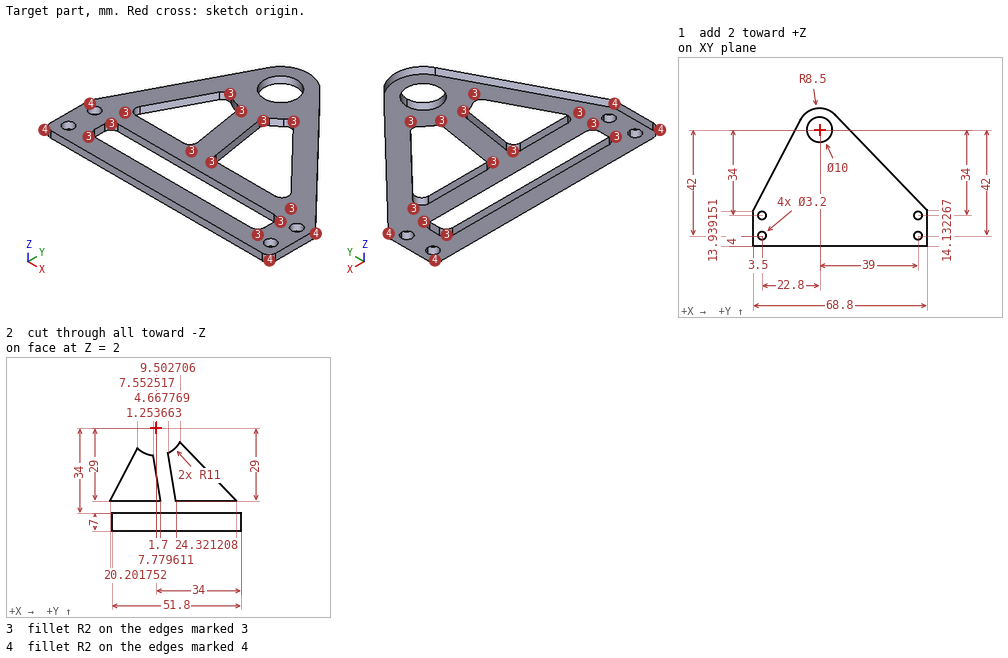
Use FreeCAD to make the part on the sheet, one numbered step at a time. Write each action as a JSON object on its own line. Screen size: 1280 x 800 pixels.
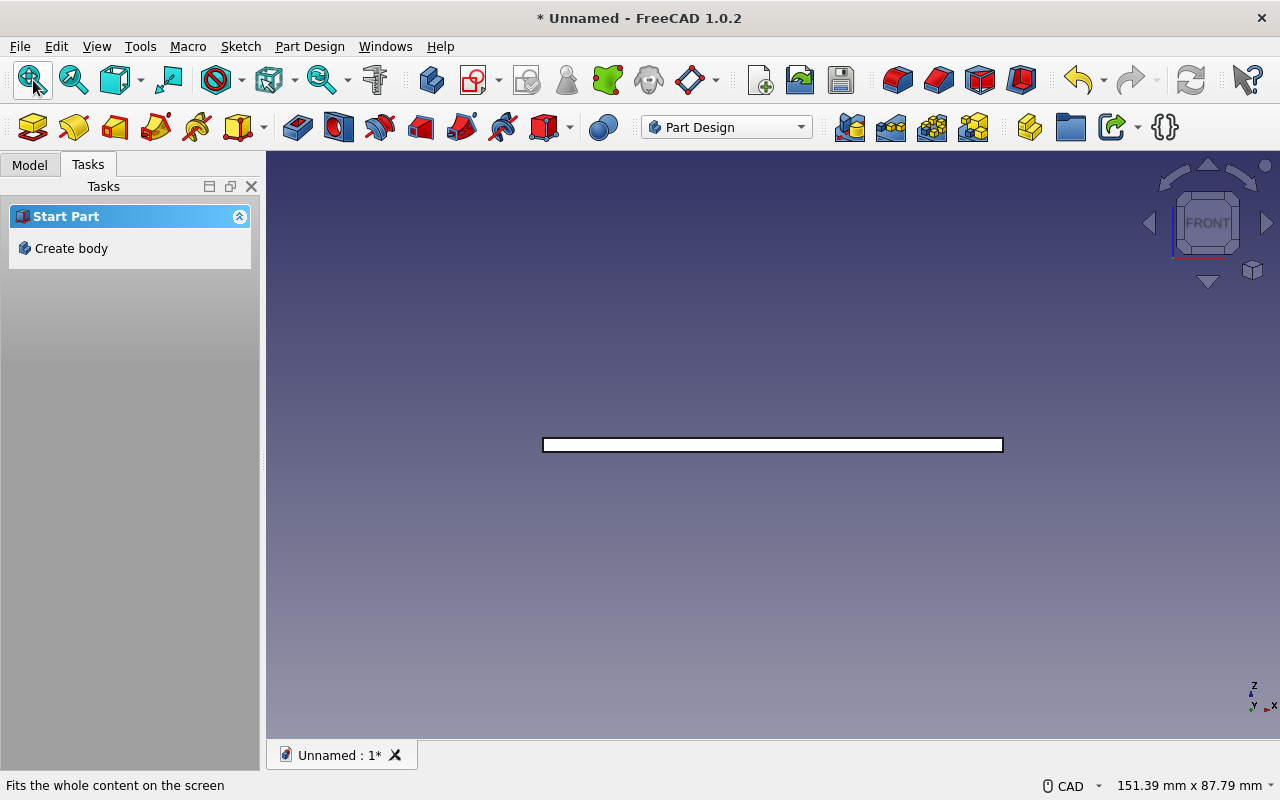
{"action": "scroll", "coordinate": [600, 444], "scroll_direction": "up", "scroll_amount": 6}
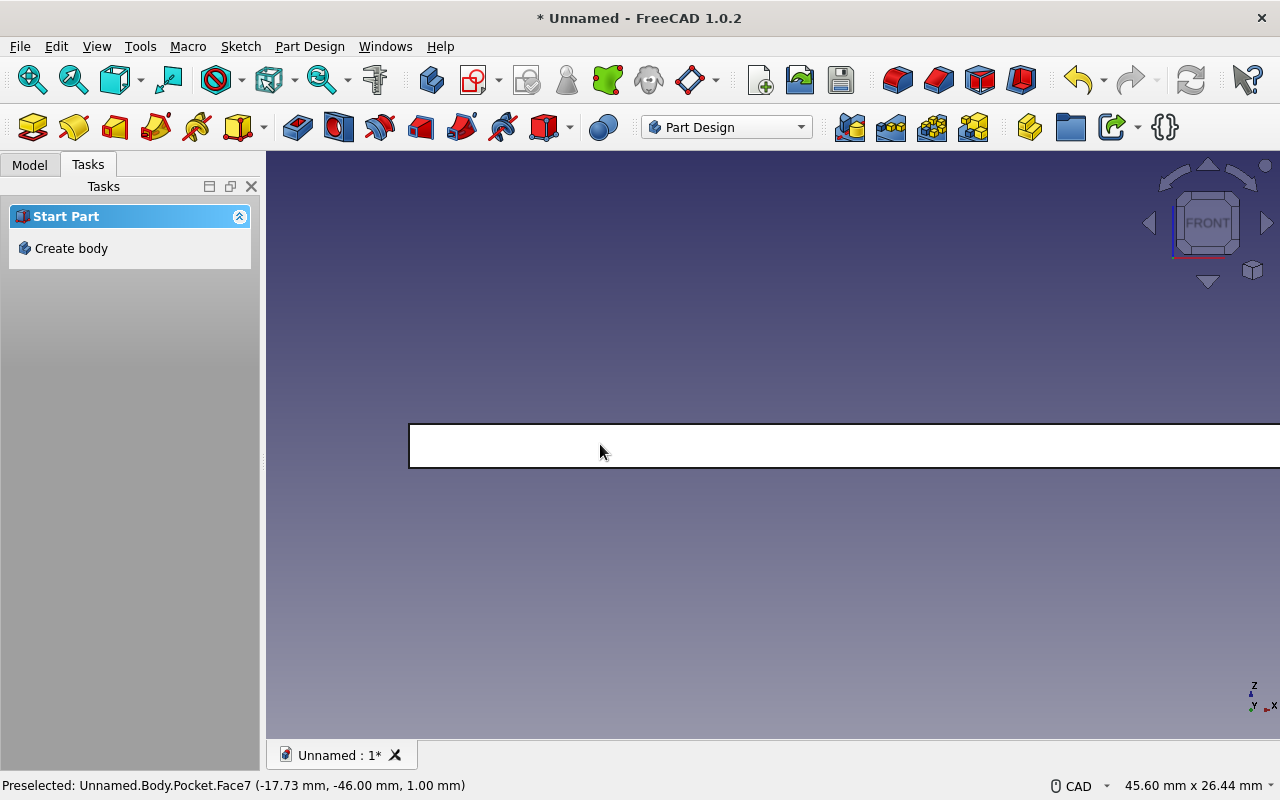
{"action": "left_click", "coordinate": [33, 80]}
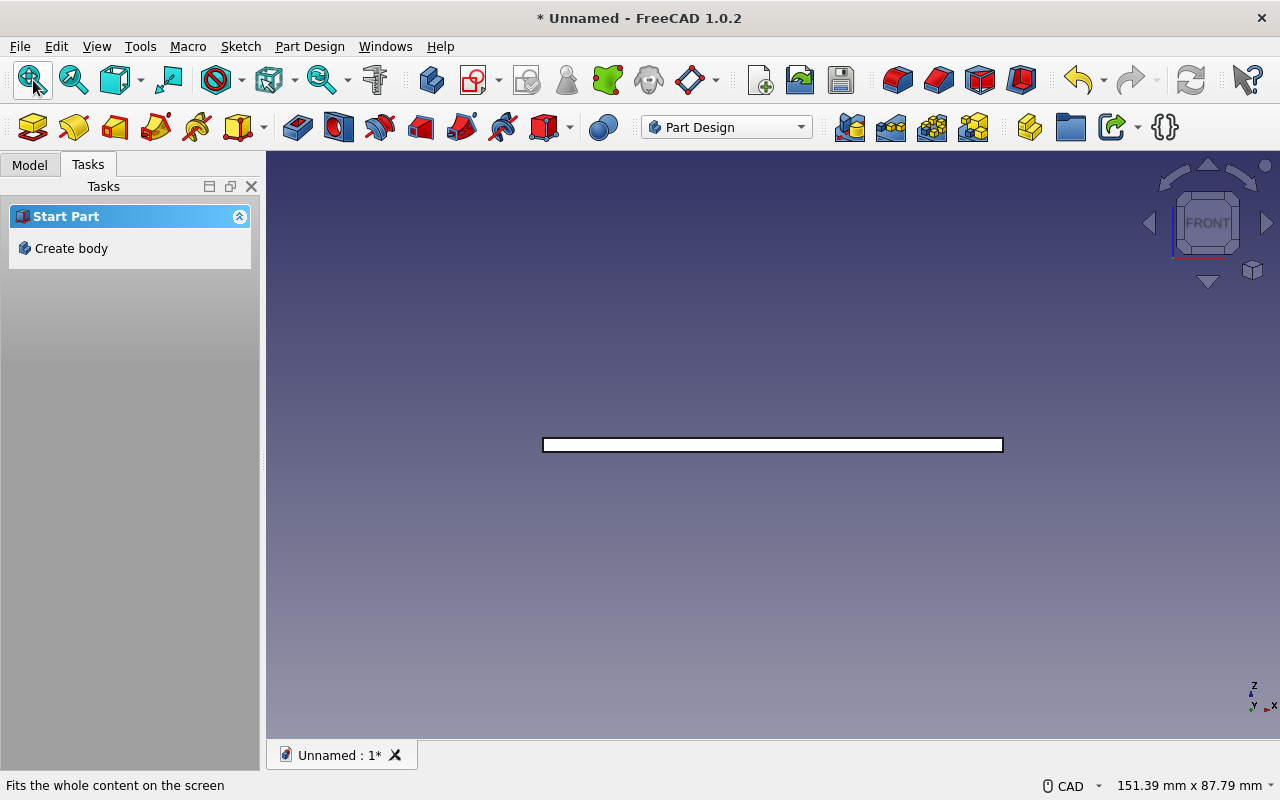
{"action": "key", "text": "3"}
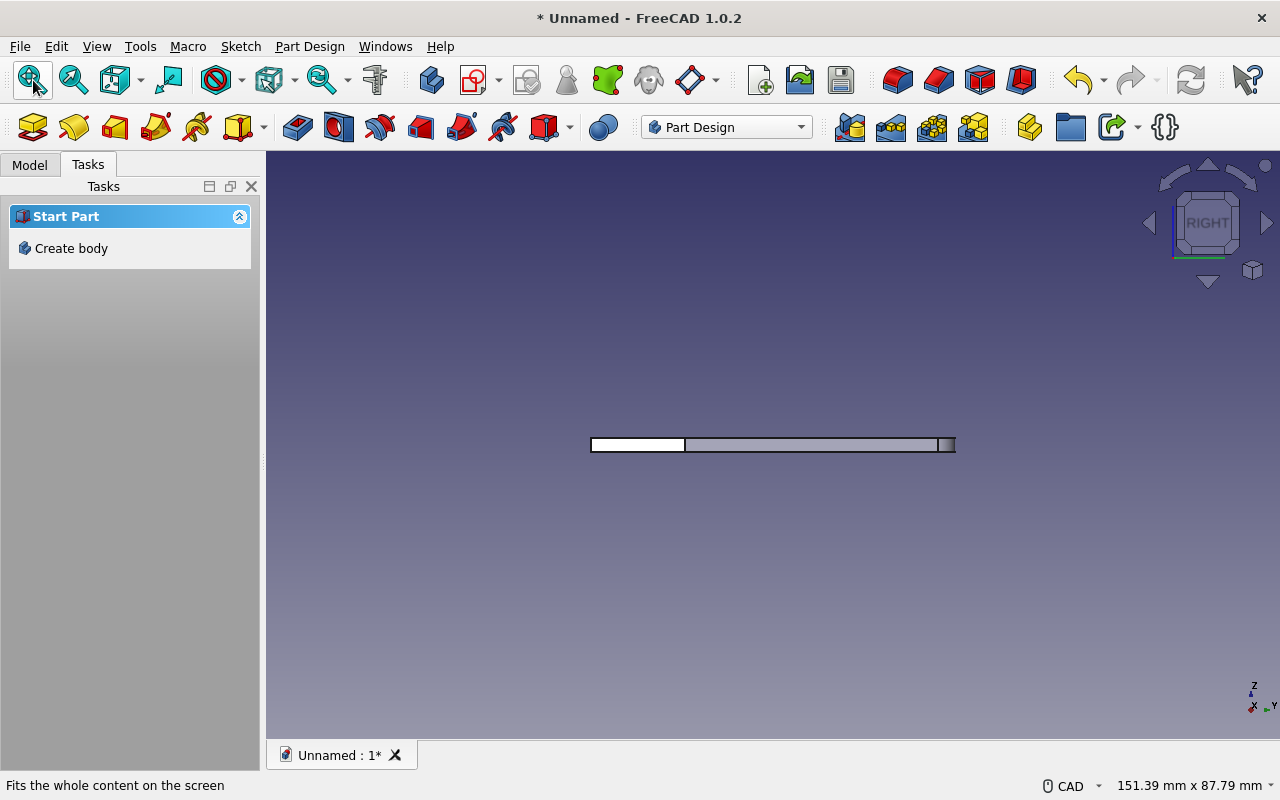
{"action": "key", "text": "v f"}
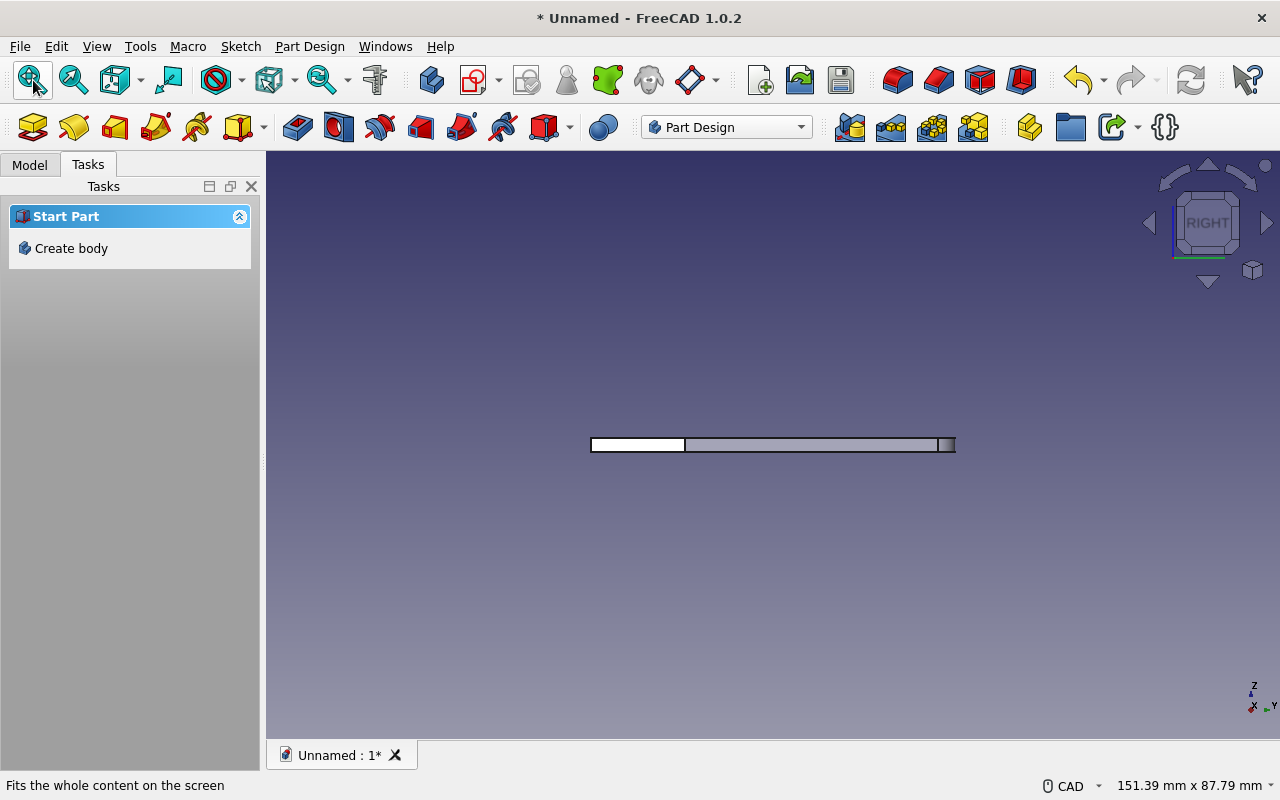
{"action": "scroll", "coordinate": [624, 444], "scroll_direction": "up", "scroll_amount": 6}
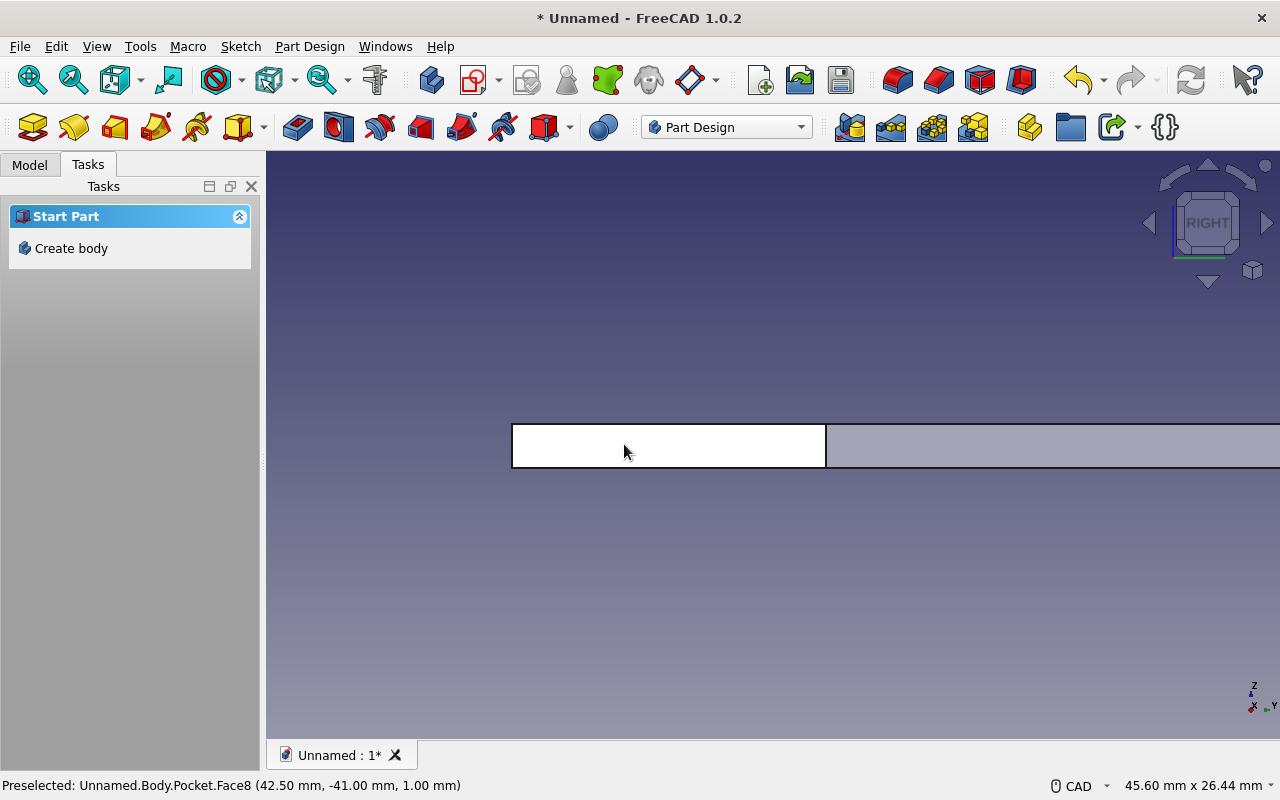
{"action": "left_click", "coordinate": [33, 80]}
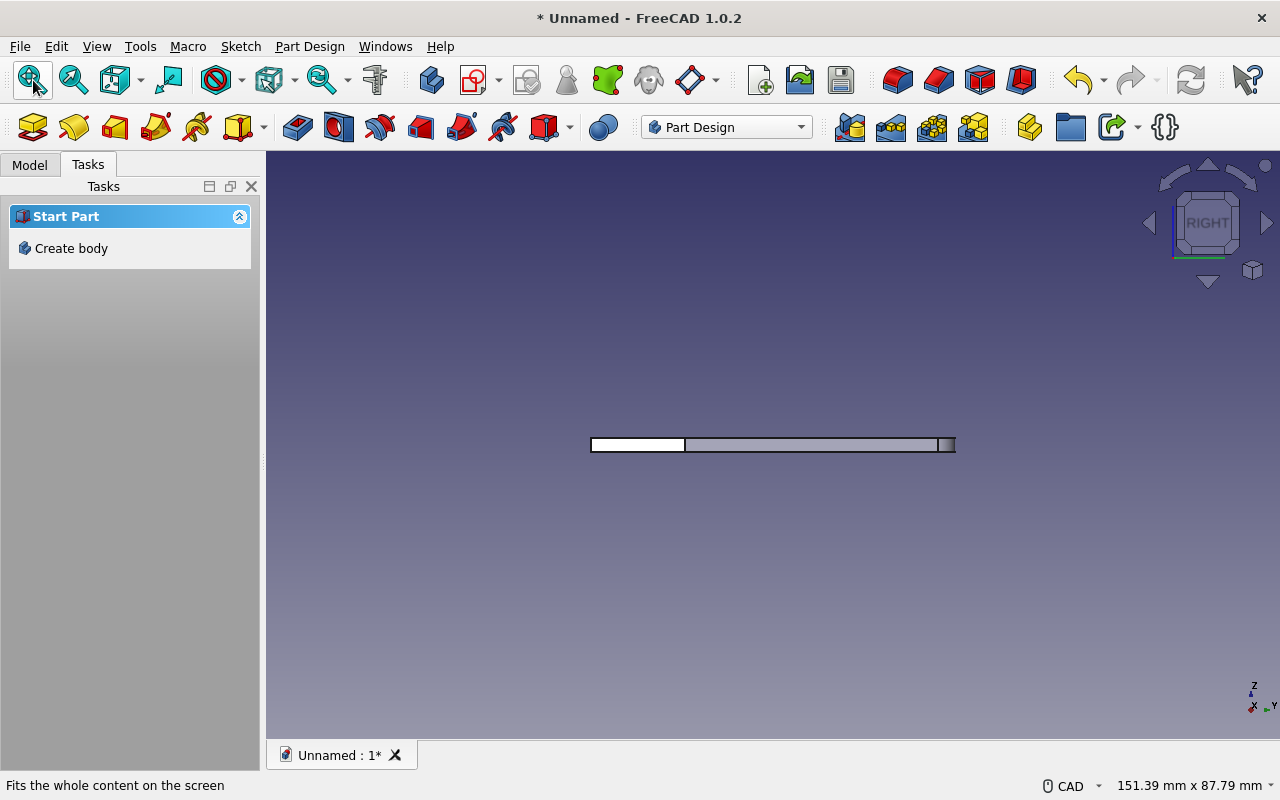
{"action": "key", "text": "5"}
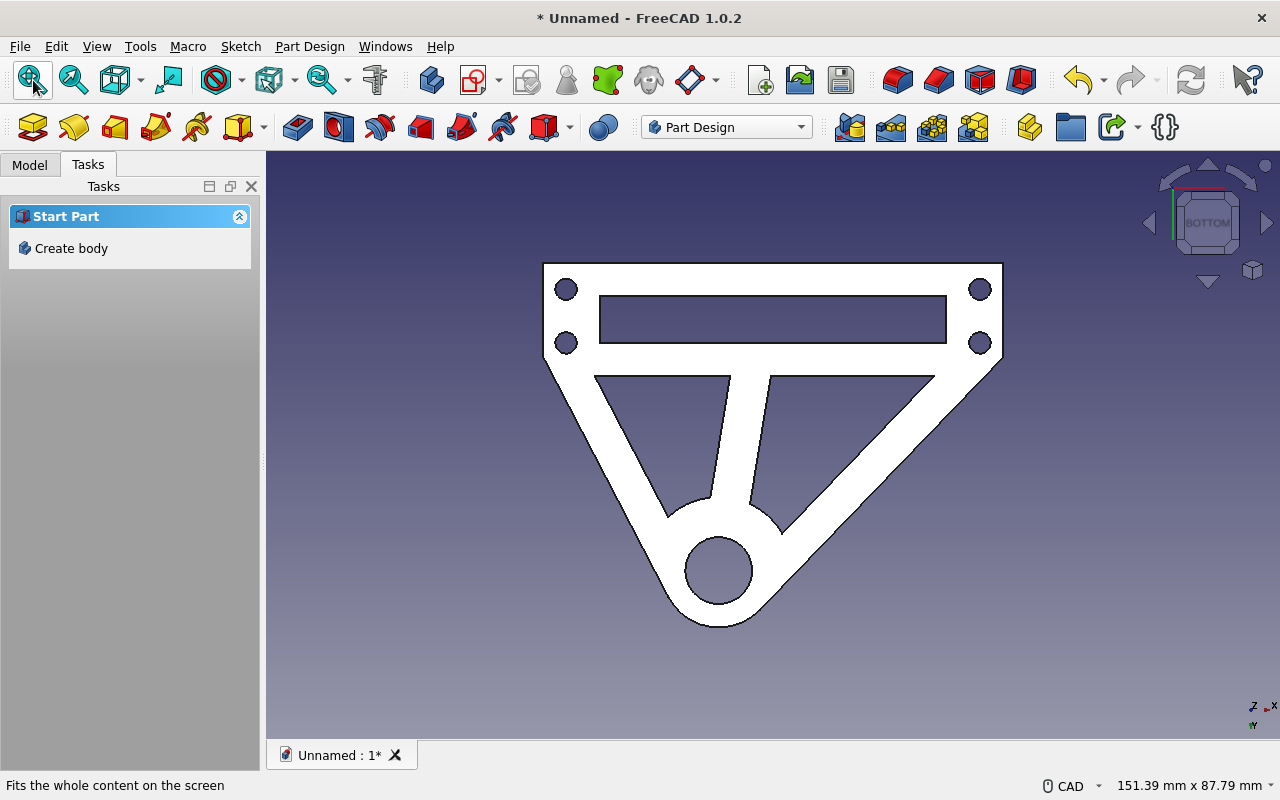
{"action": "scroll", "coordinate": [600, 295], "scroll_direction": "up", "scroll_amount": 6}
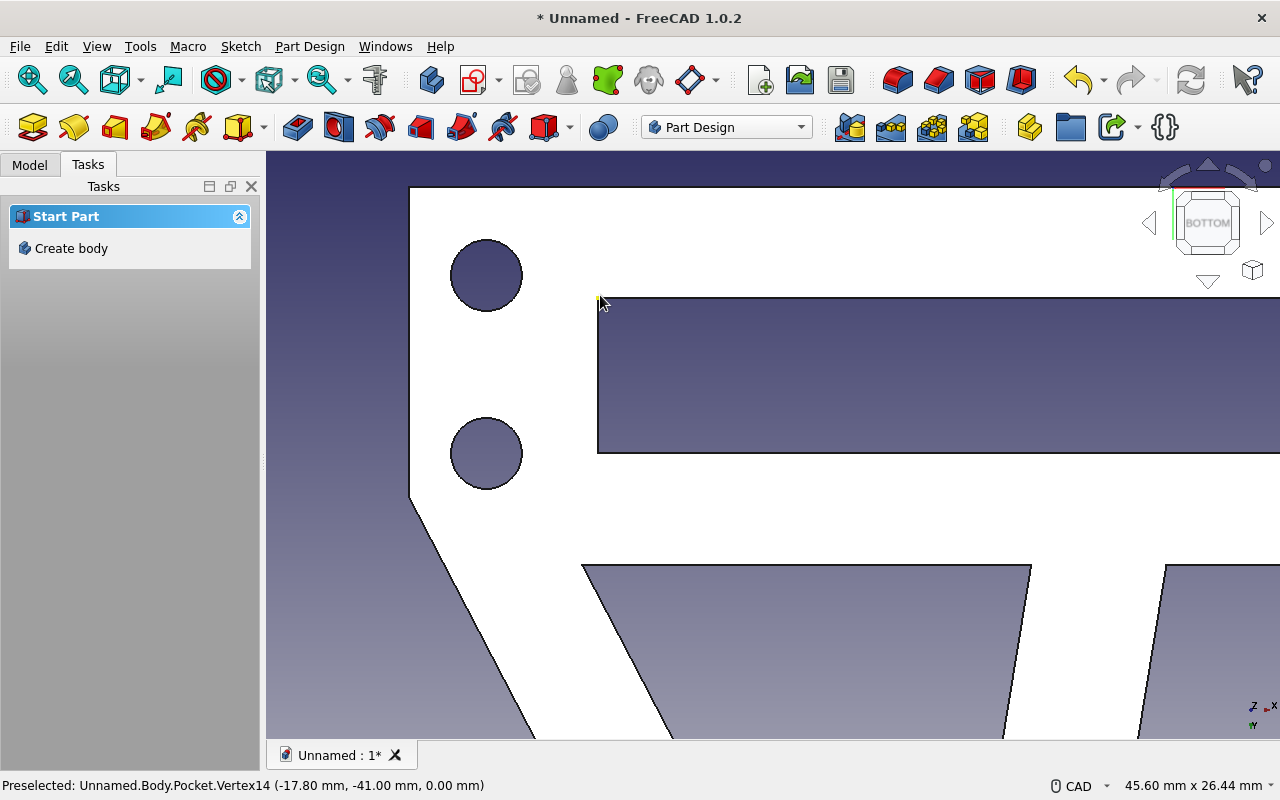
{"action": "key", "text": "v f"}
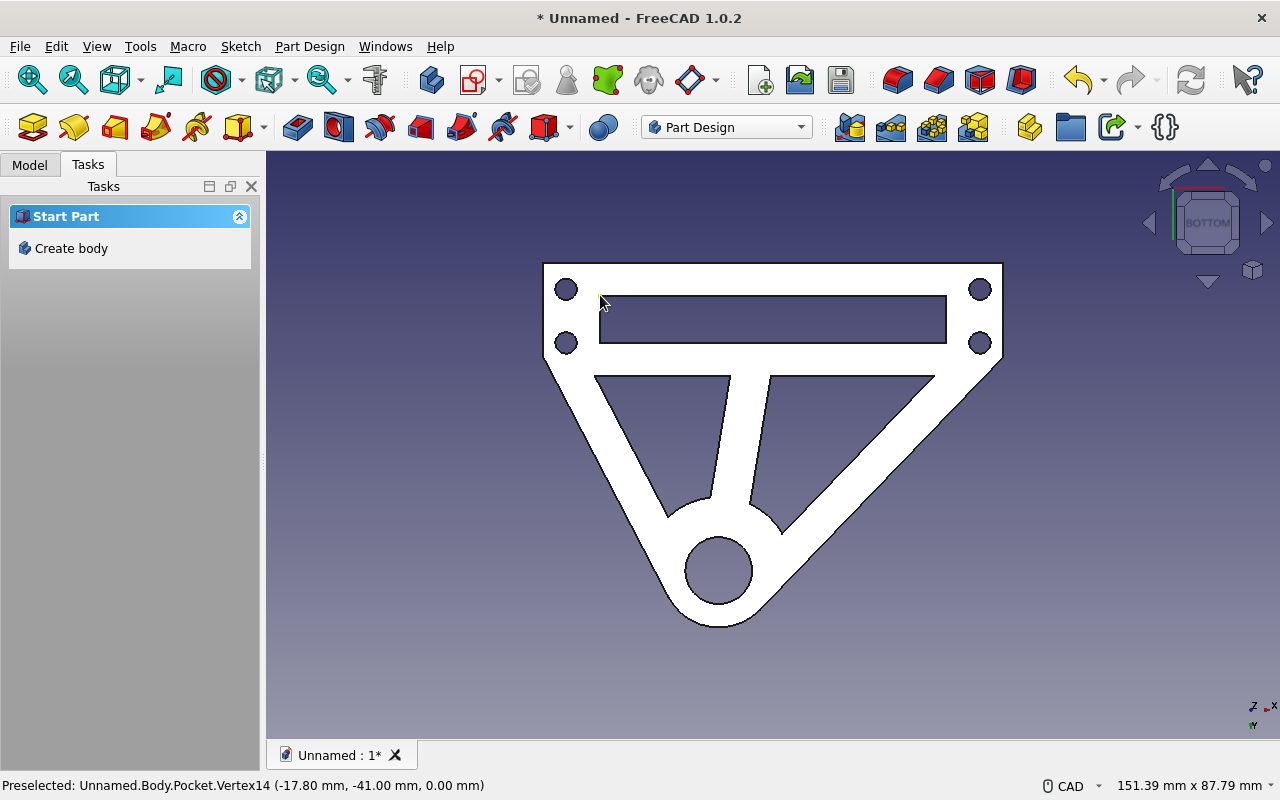
{"action": "key", "text": "4"}